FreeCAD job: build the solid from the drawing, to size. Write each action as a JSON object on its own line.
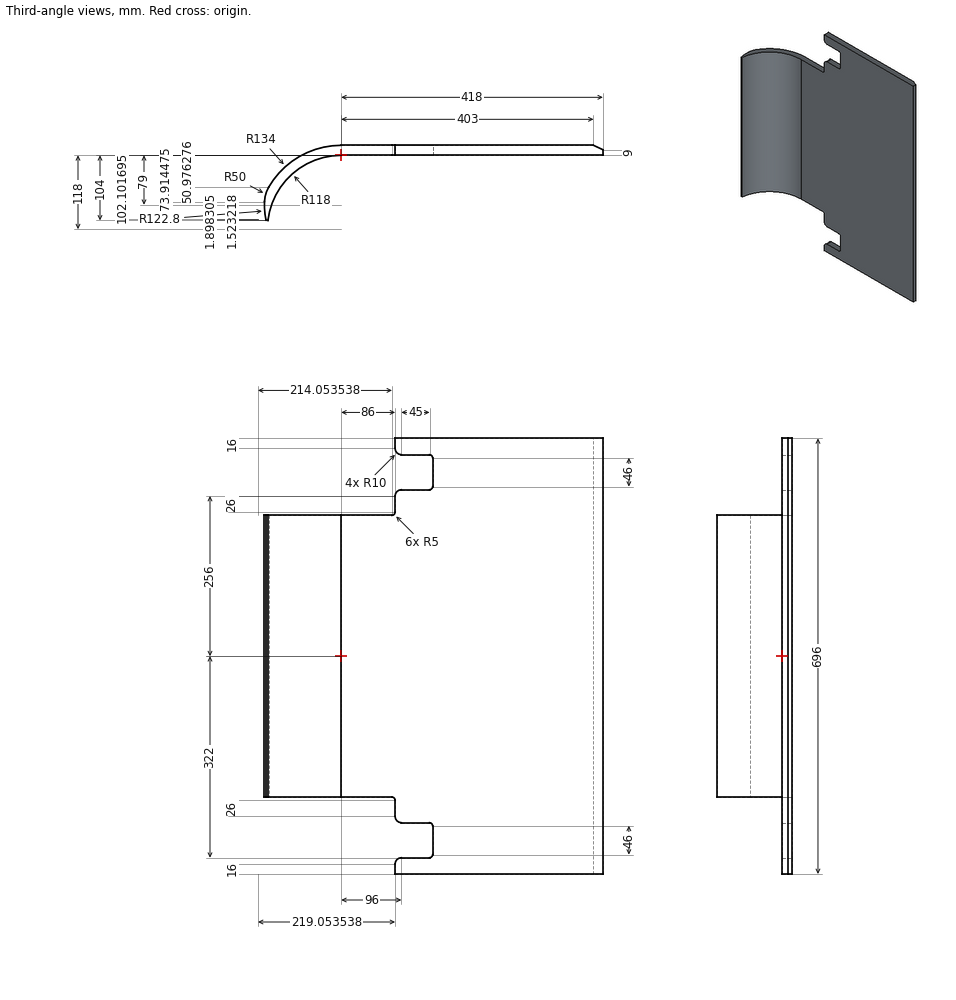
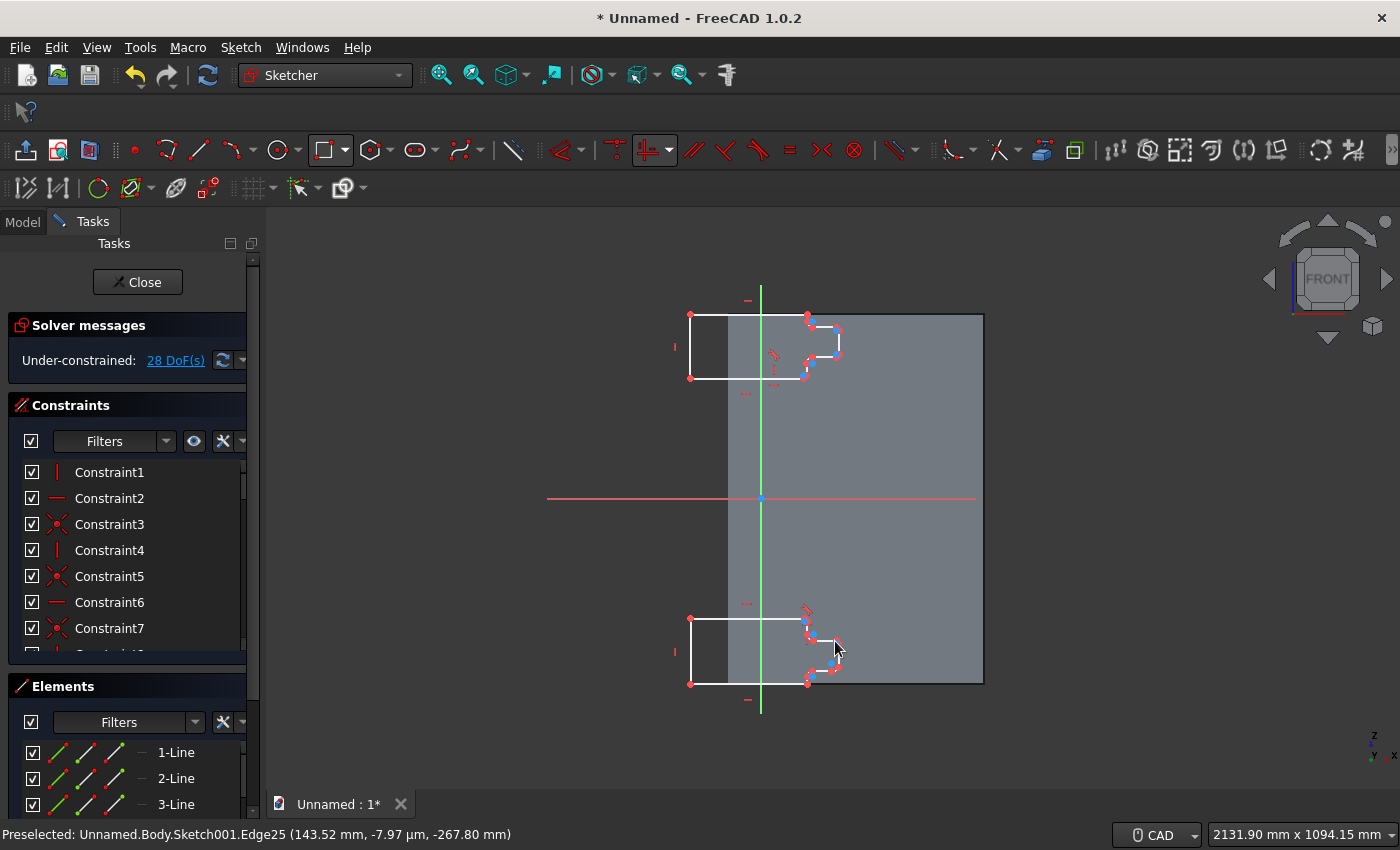
{"action": "scroll", "coordinate": [839, 650], "scroll_direction": "up", "scroll_amount": 4}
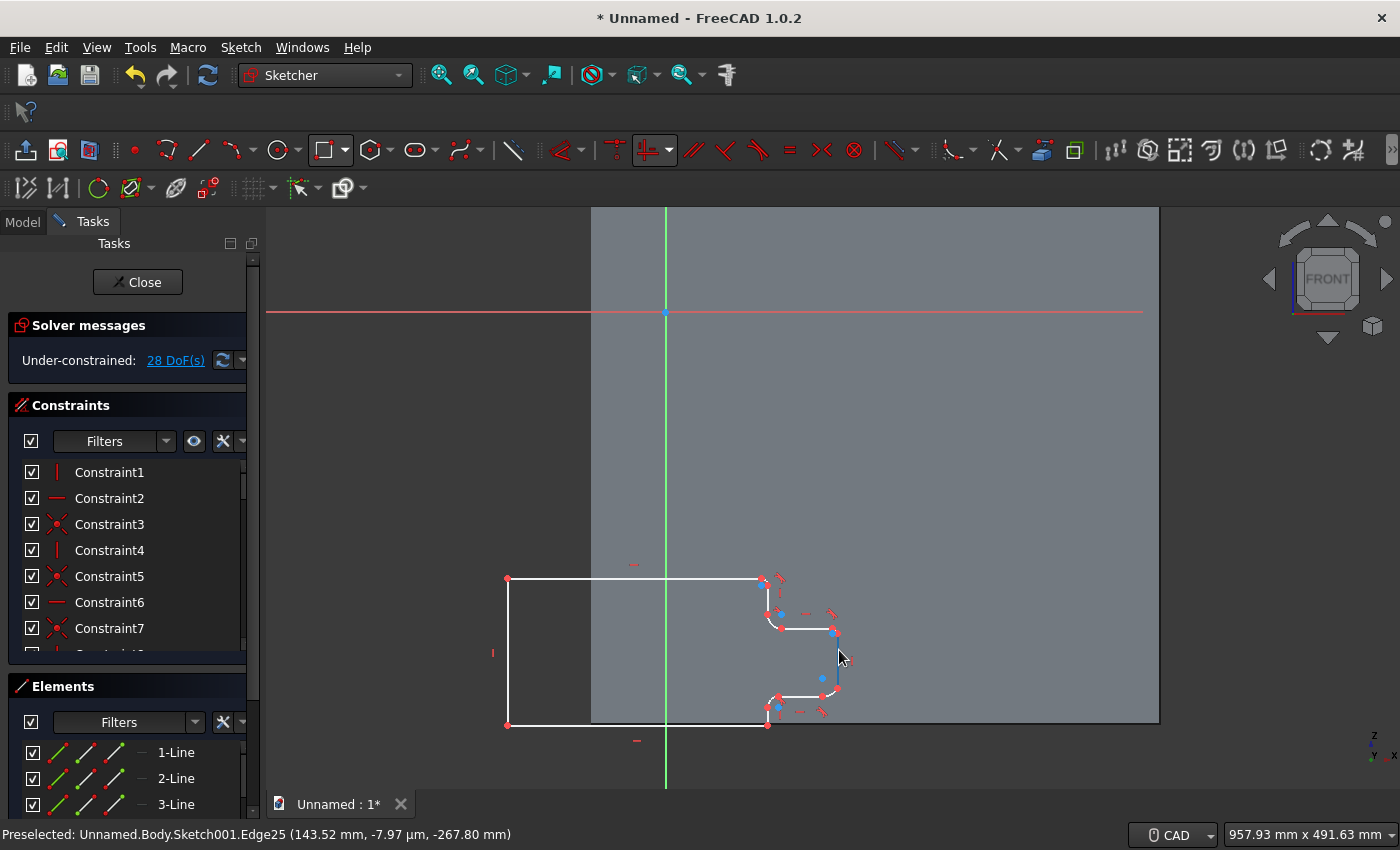
{"action": "left_click", "coordinate": [838, 650]}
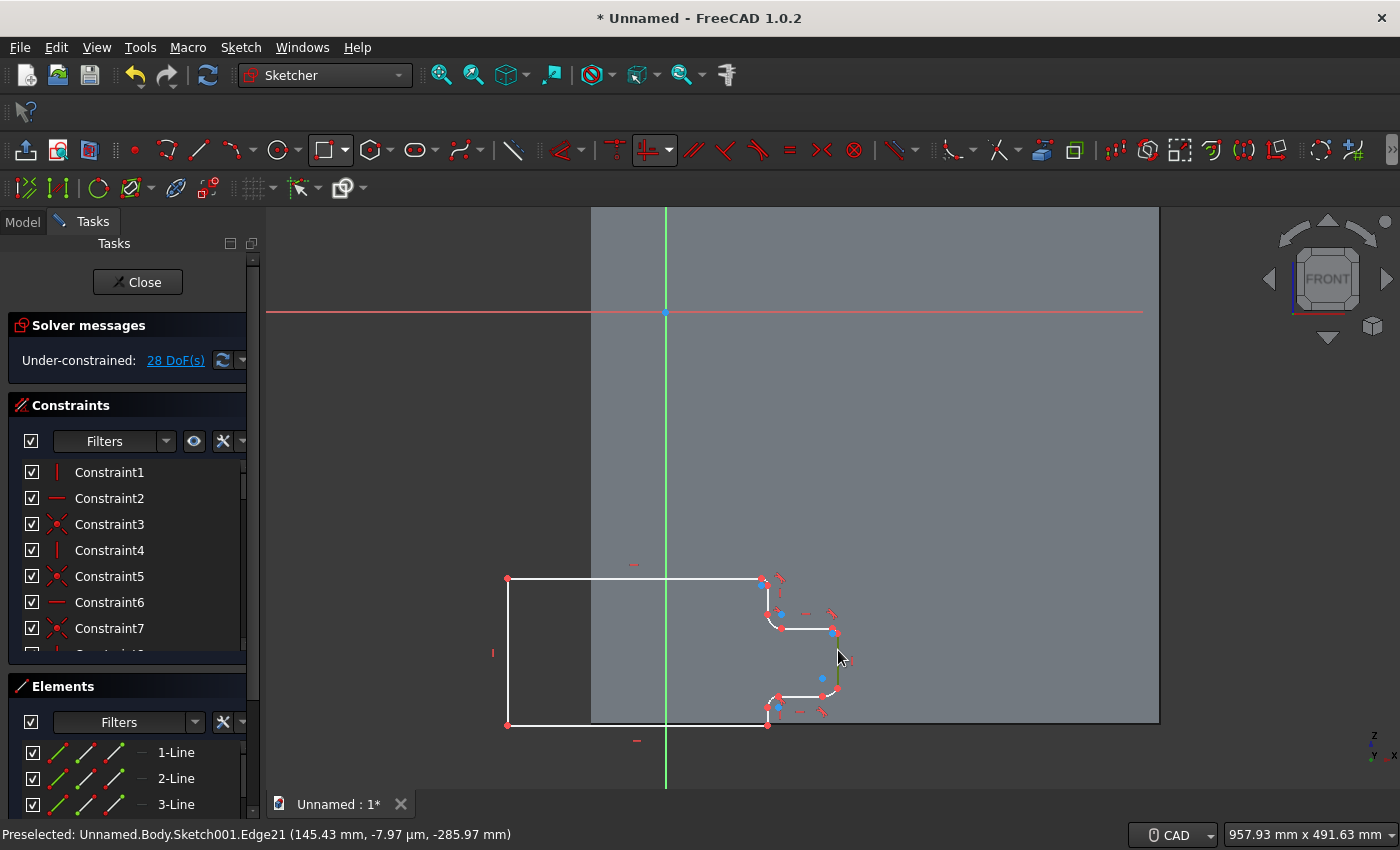
{"action": "scroll", "coordinate": [836, 630], "scroll_direction": "up", "scroll_amount": 7}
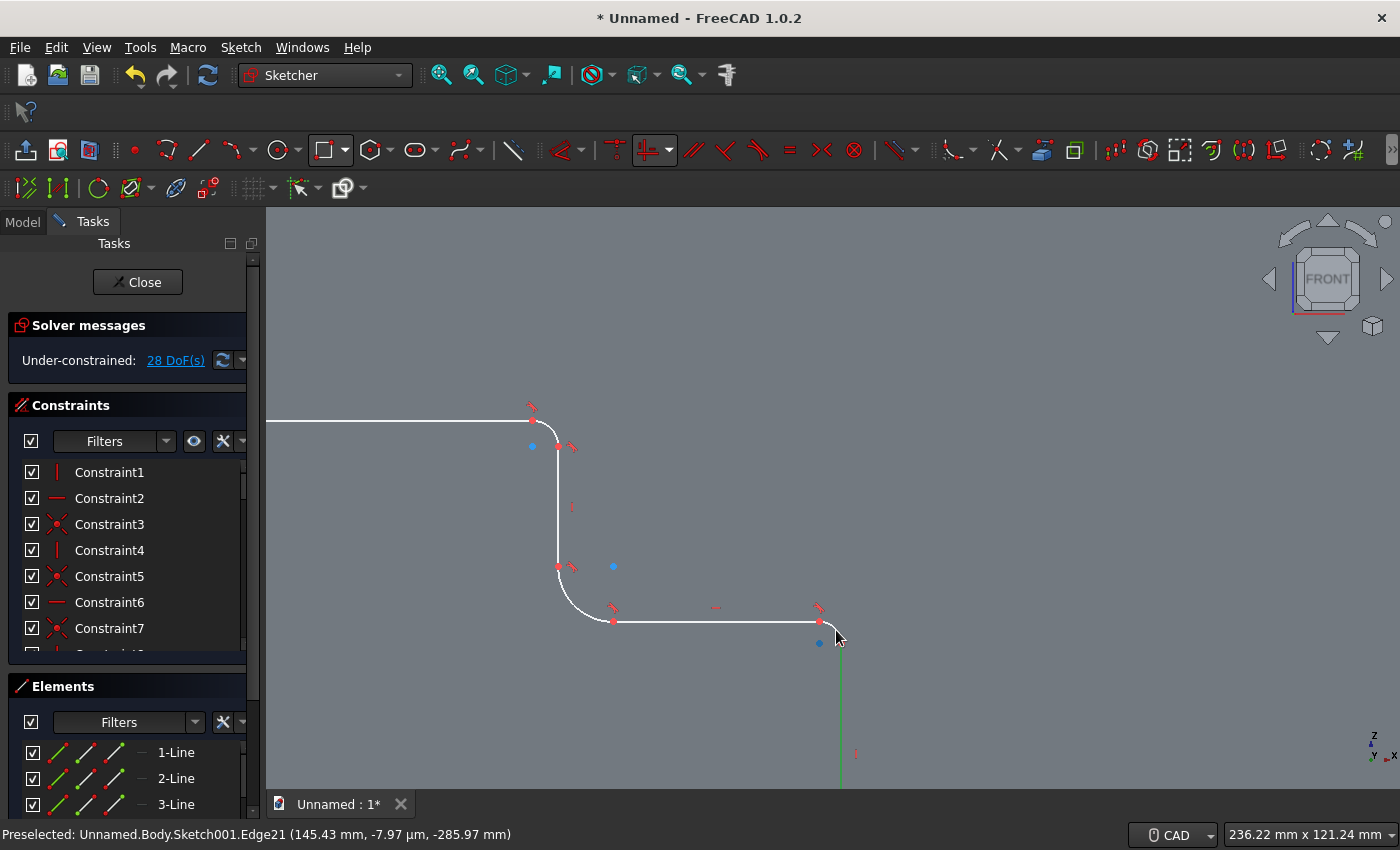
{"action": "left_click", "coordinate": [835, 628]}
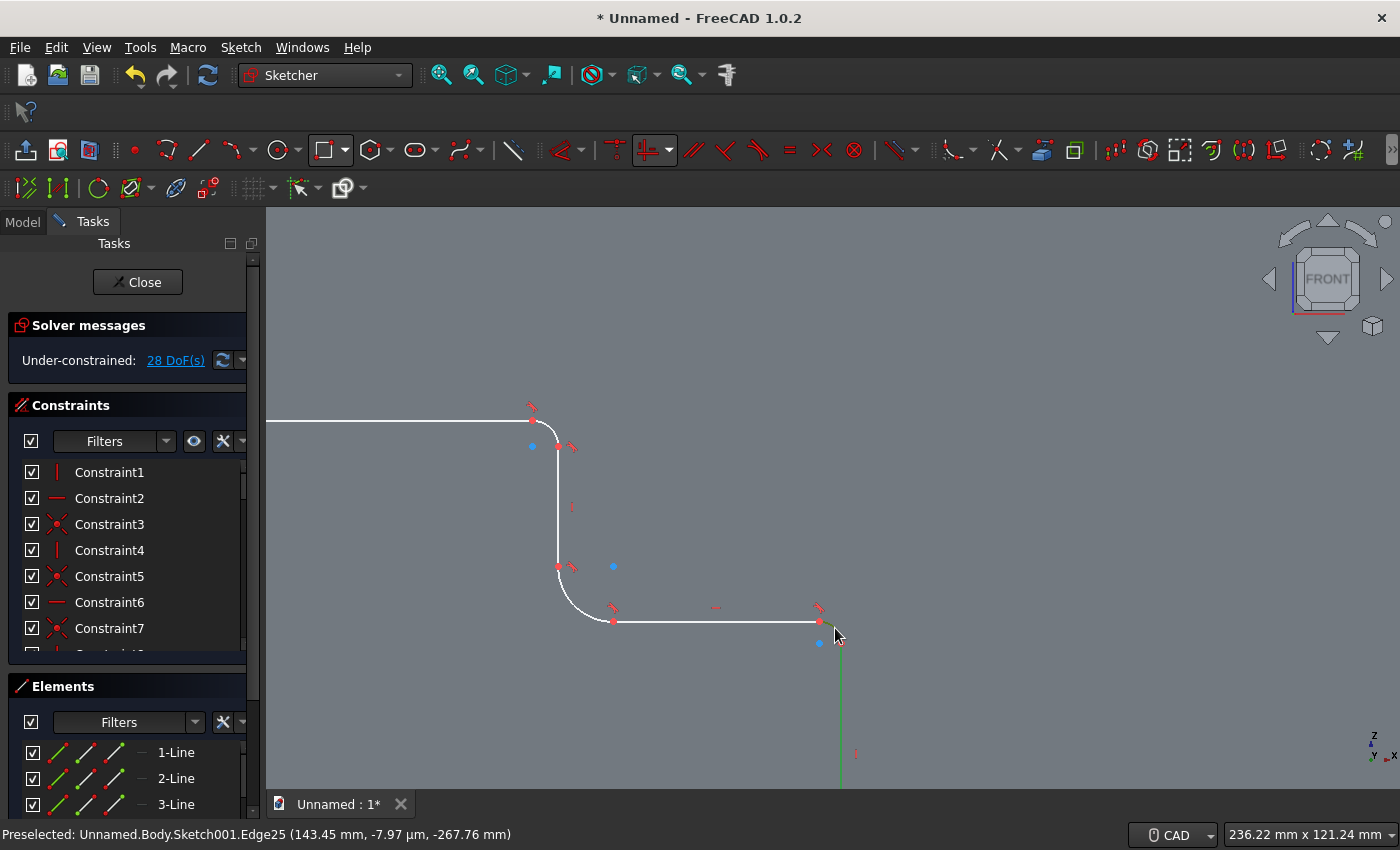
{"action": "left_click", "coordinate": [758, 150]}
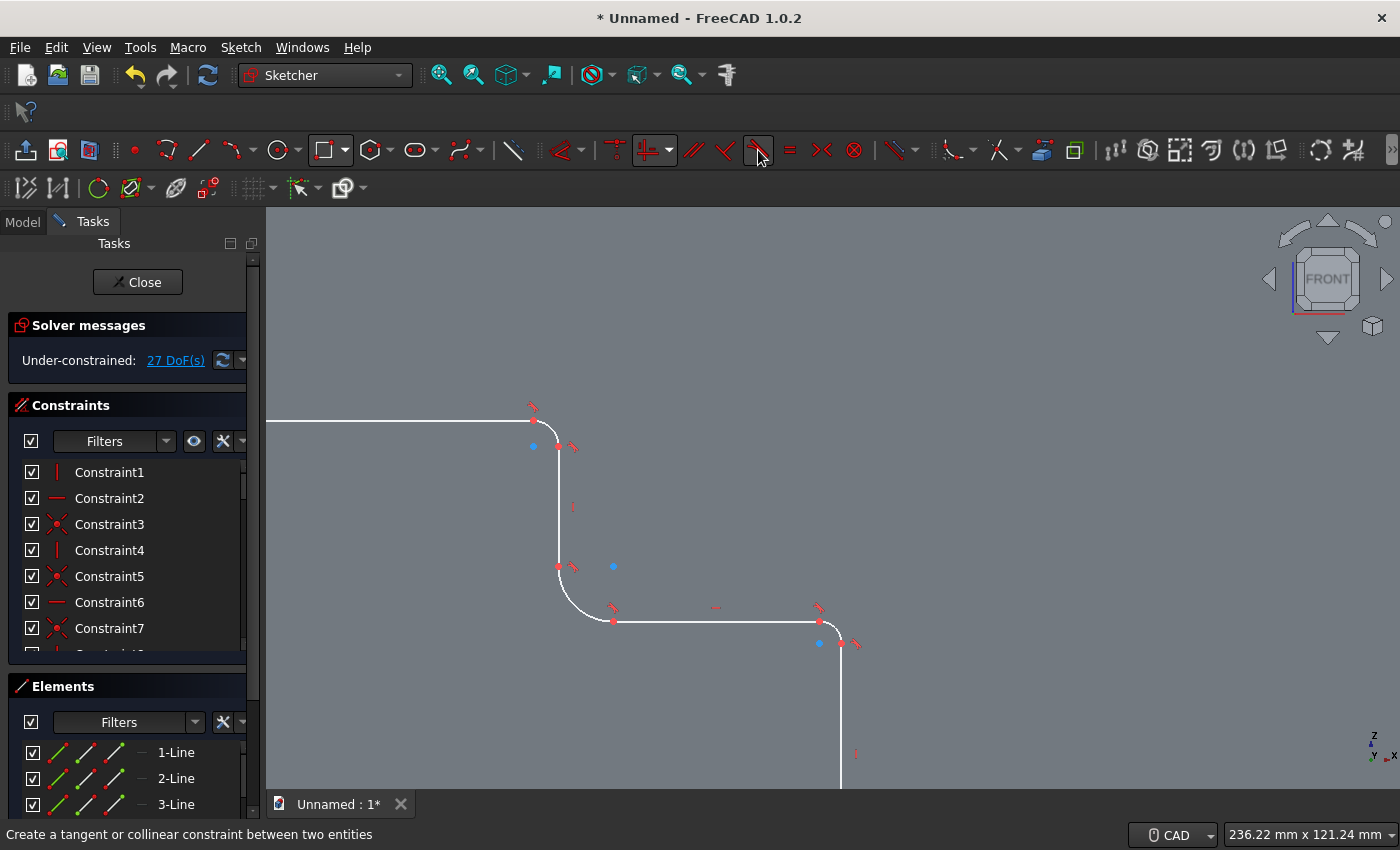
{"action": "scroll", "coordinate": [838, 642], "scroll_direction": "down", "scroll_amount": 11}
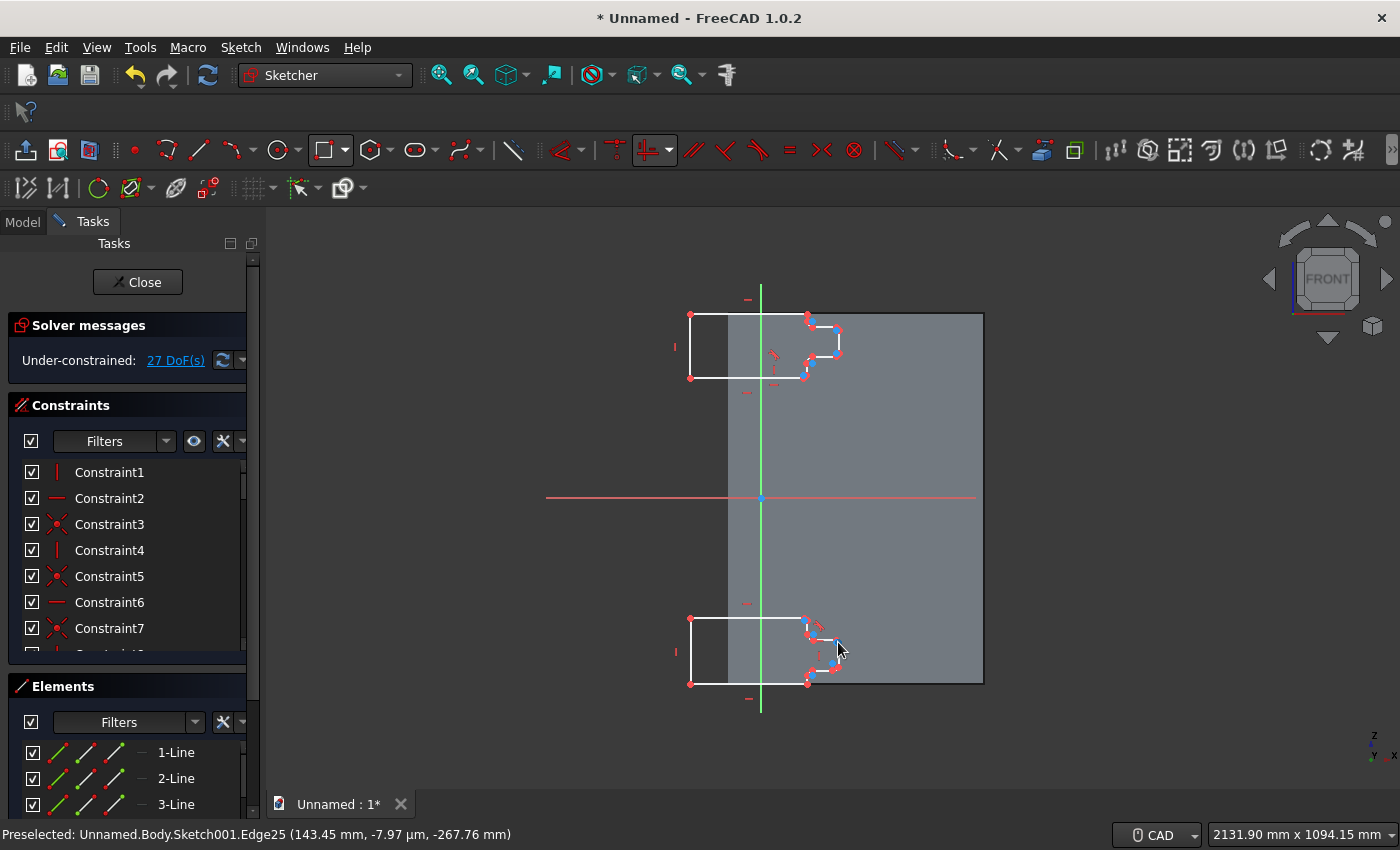
{"action": "scroll", "coordinate": [839, 650], "scroll_direction": "up", "scroll_amount": 4}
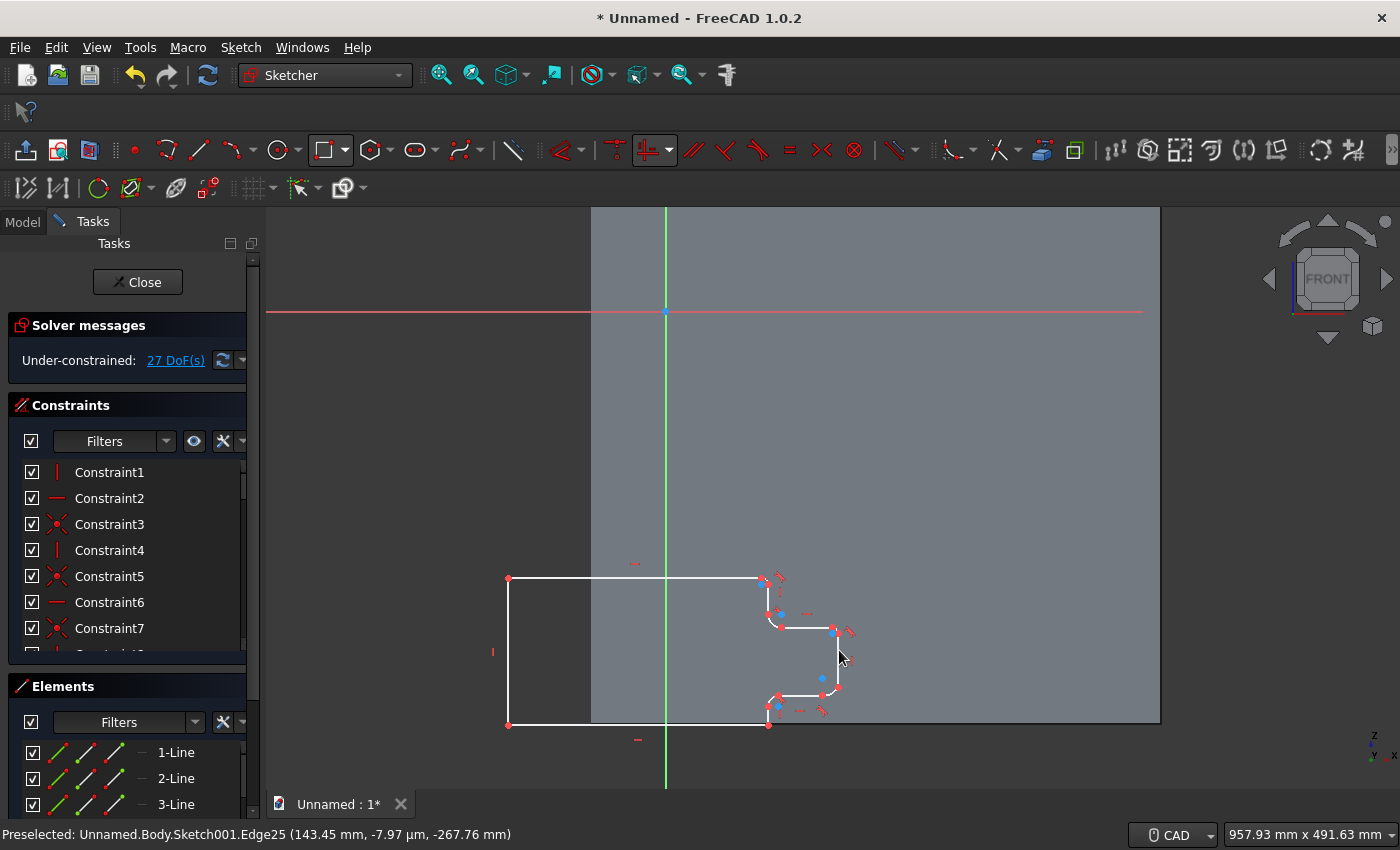
{"action": "left_click", "coordinate": [838, 649]}